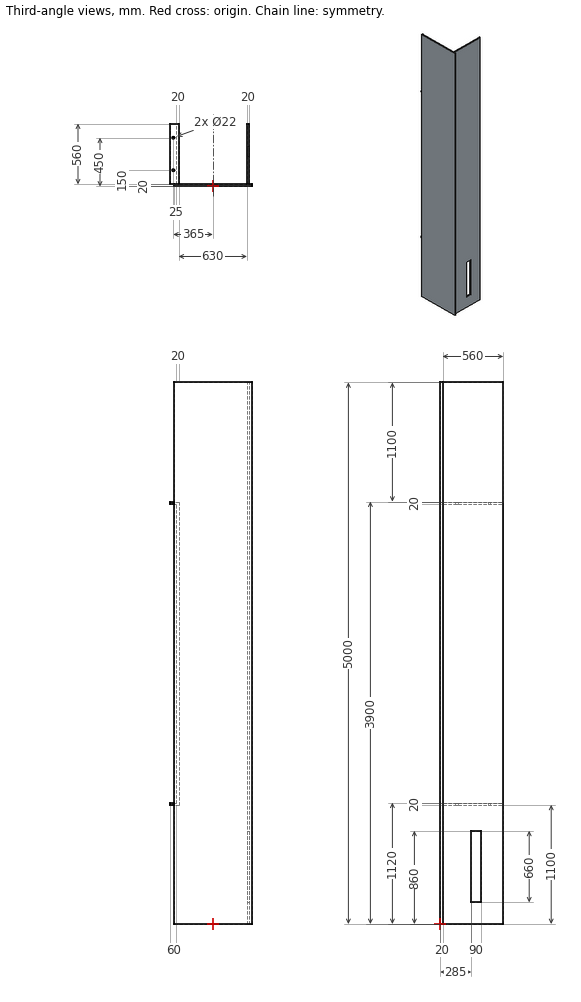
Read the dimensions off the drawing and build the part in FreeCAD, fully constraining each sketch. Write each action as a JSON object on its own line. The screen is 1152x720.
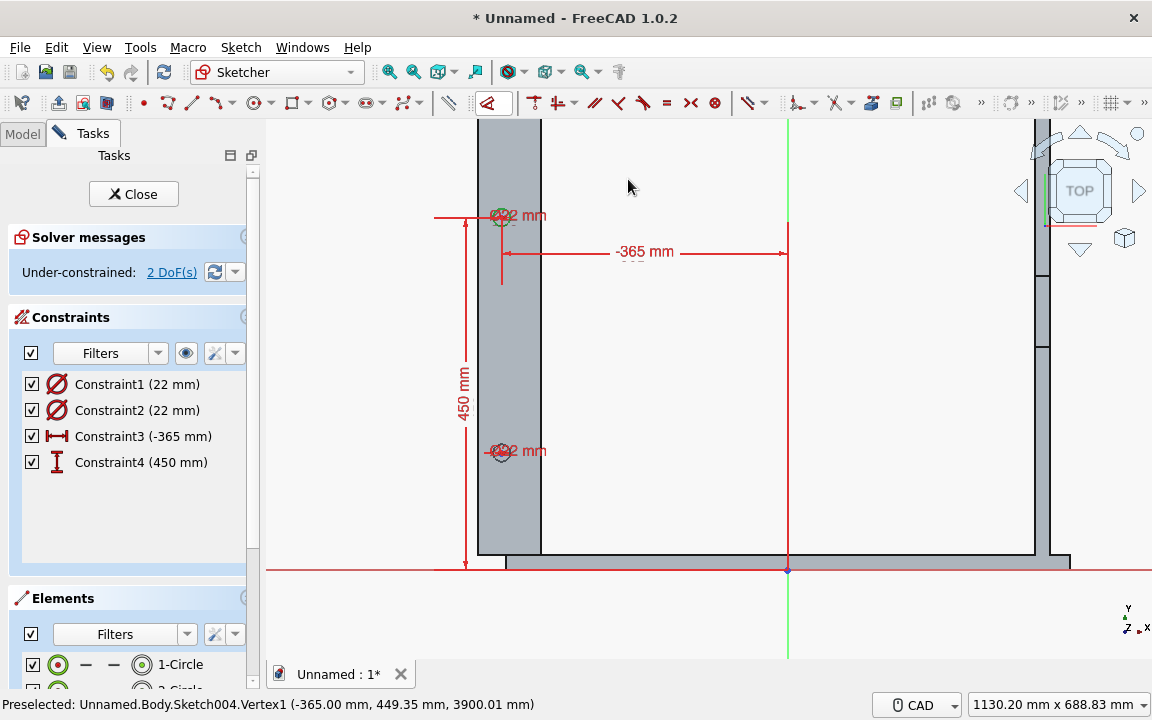
{"action": "left_click", "coordinate": [502, 453]}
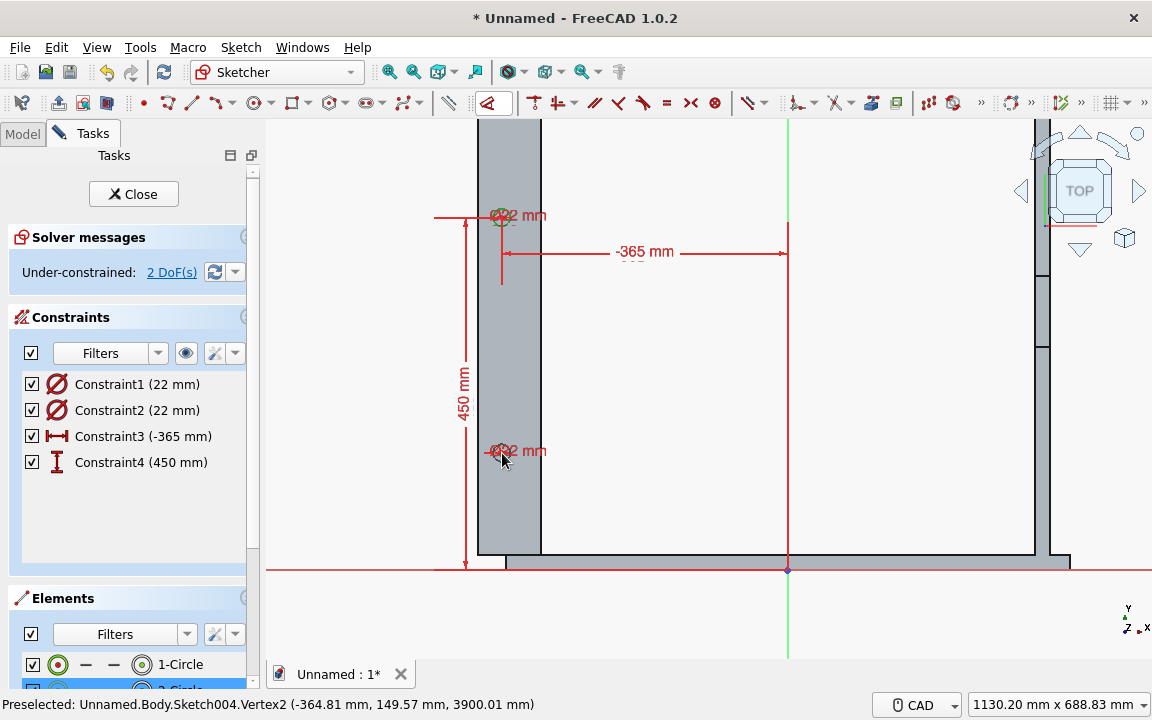
{"action": "key", "text": "l"}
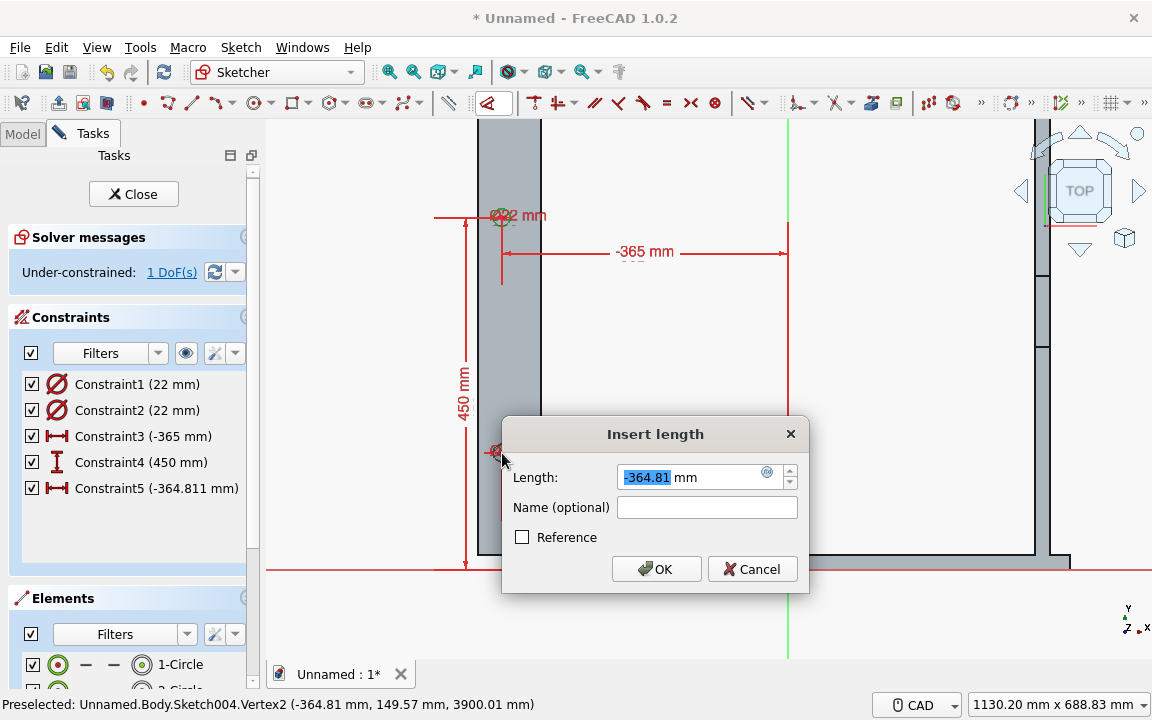
{"action": "type", "text": "-365"}
{"action": "key", "text": "Return"}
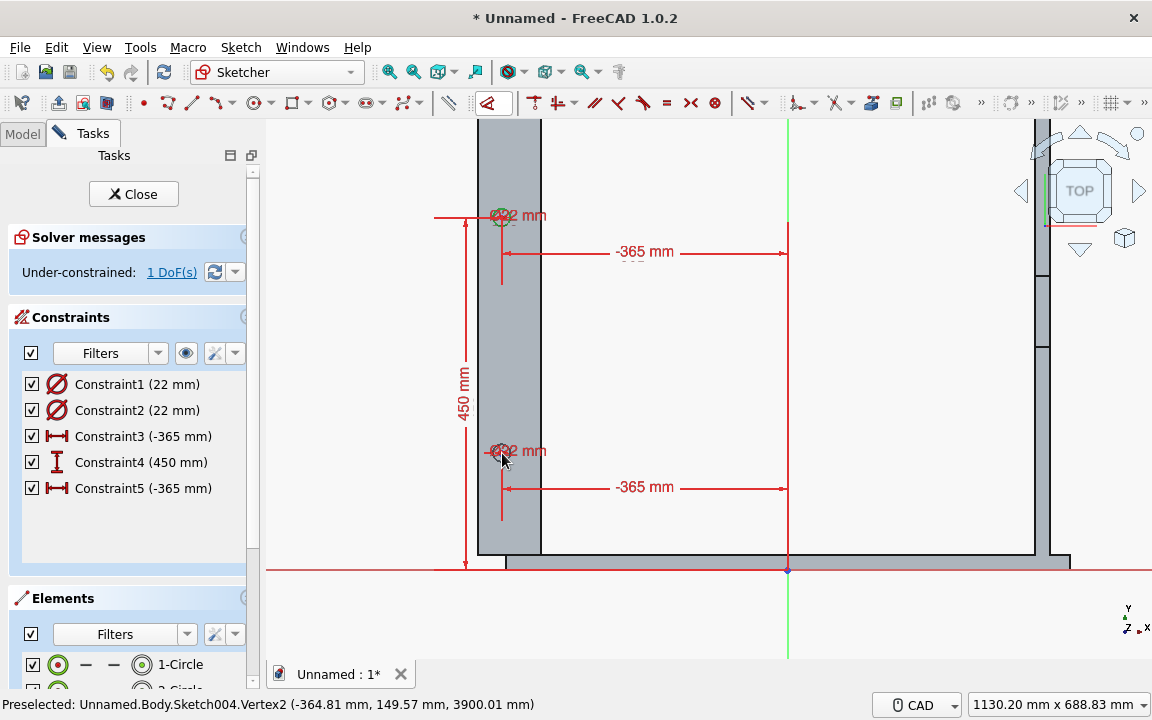
{"action": "left_click", "coordinate": [502, 453]}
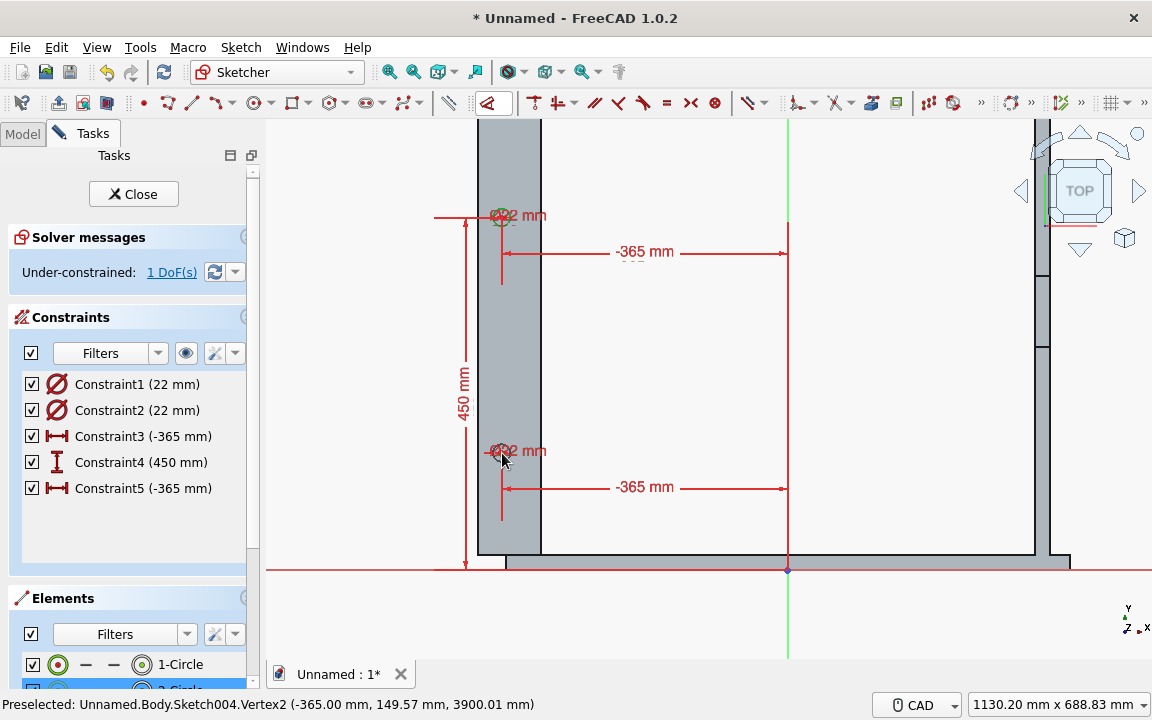
{"action": "left_click", "coordinate": [506, 104]}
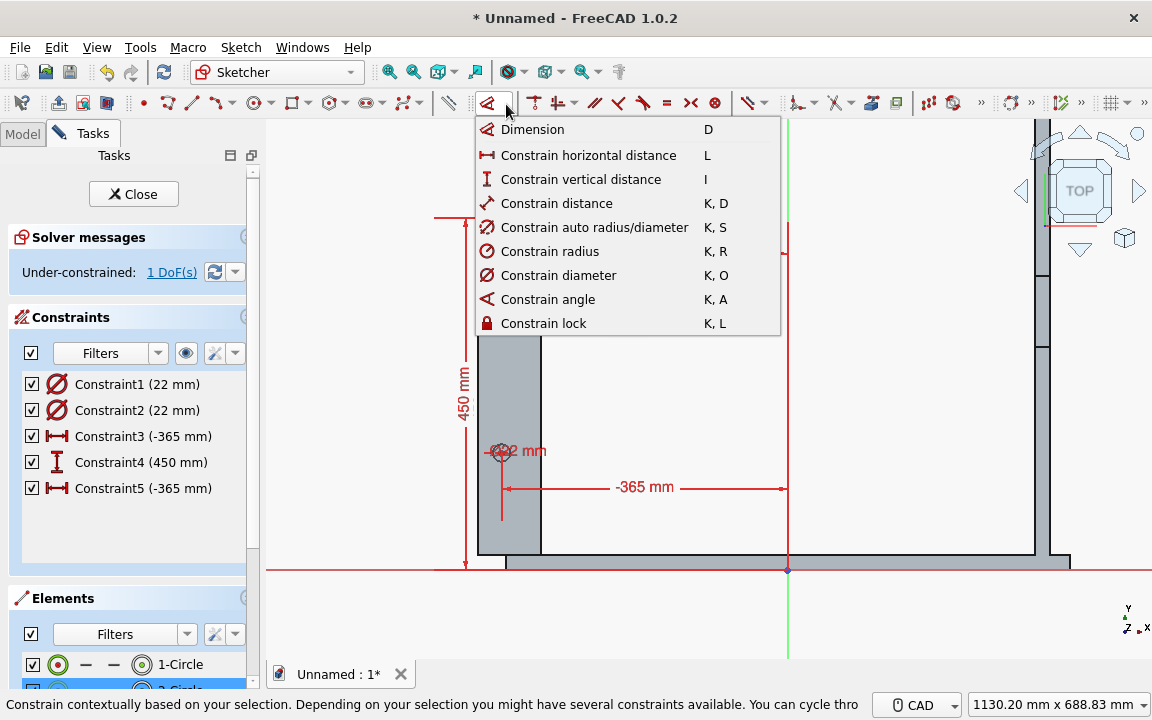
{"action": "left_click", "coordinate": [628, 179]}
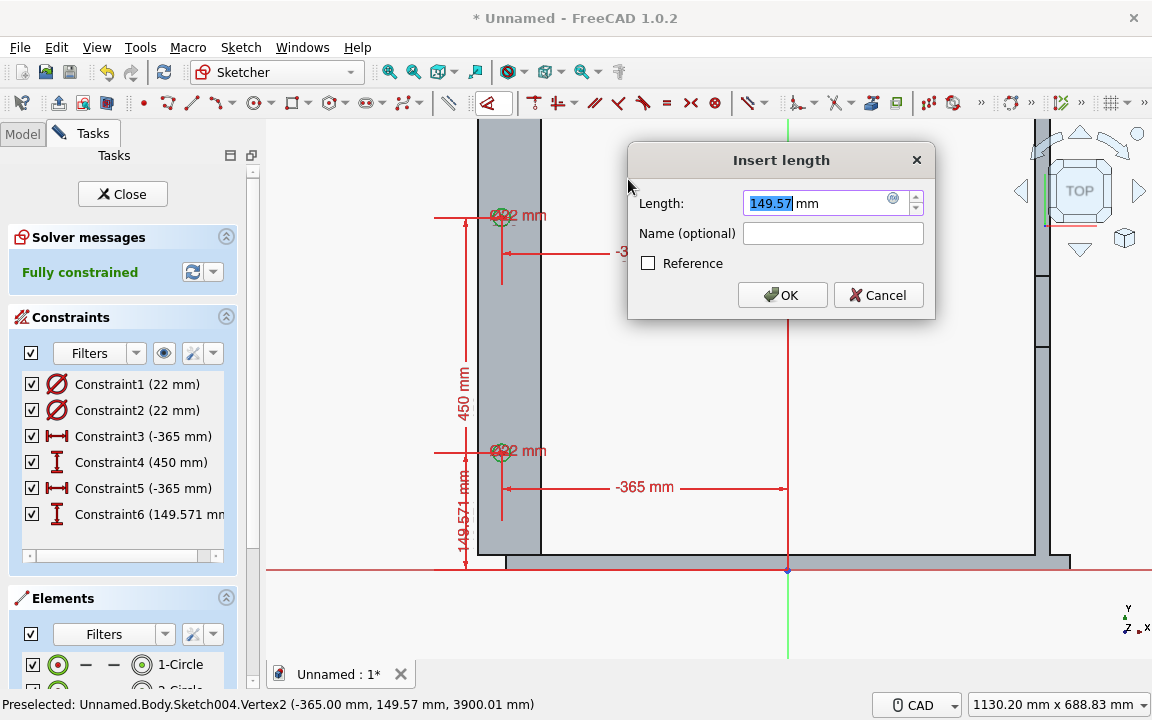
{"action": "type", "text": "150"}
{"action": "key", "text": "Return"}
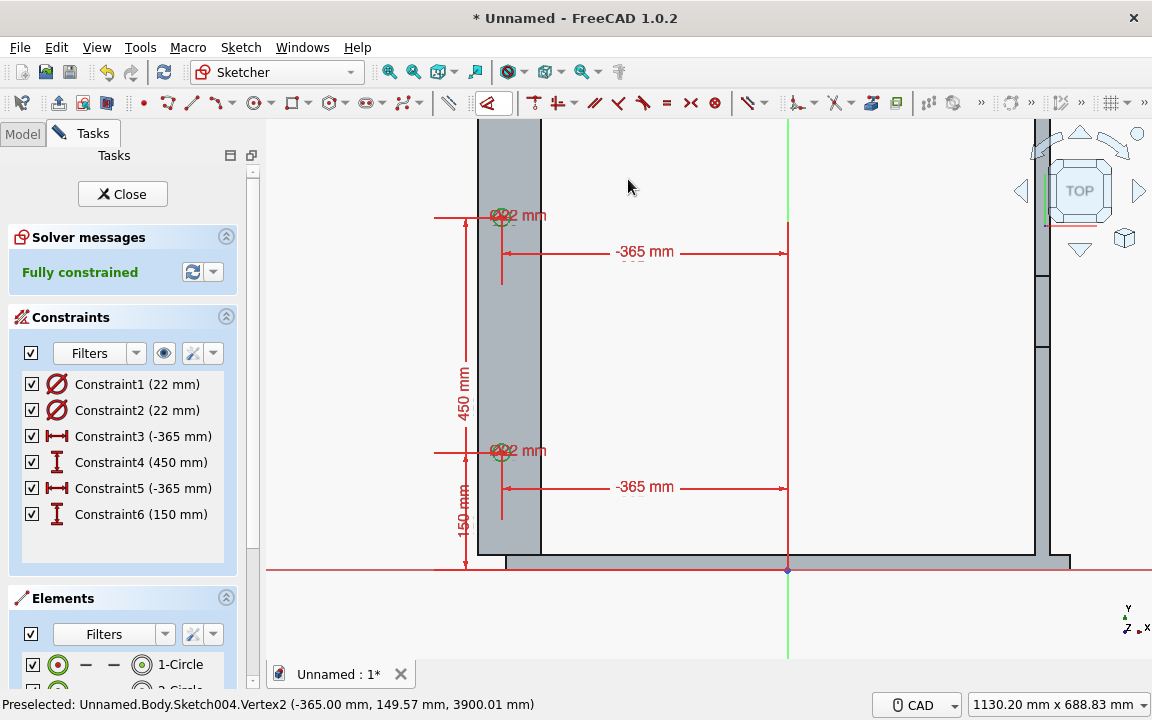
{"action": "left_click", "coordinate": [123, 194]}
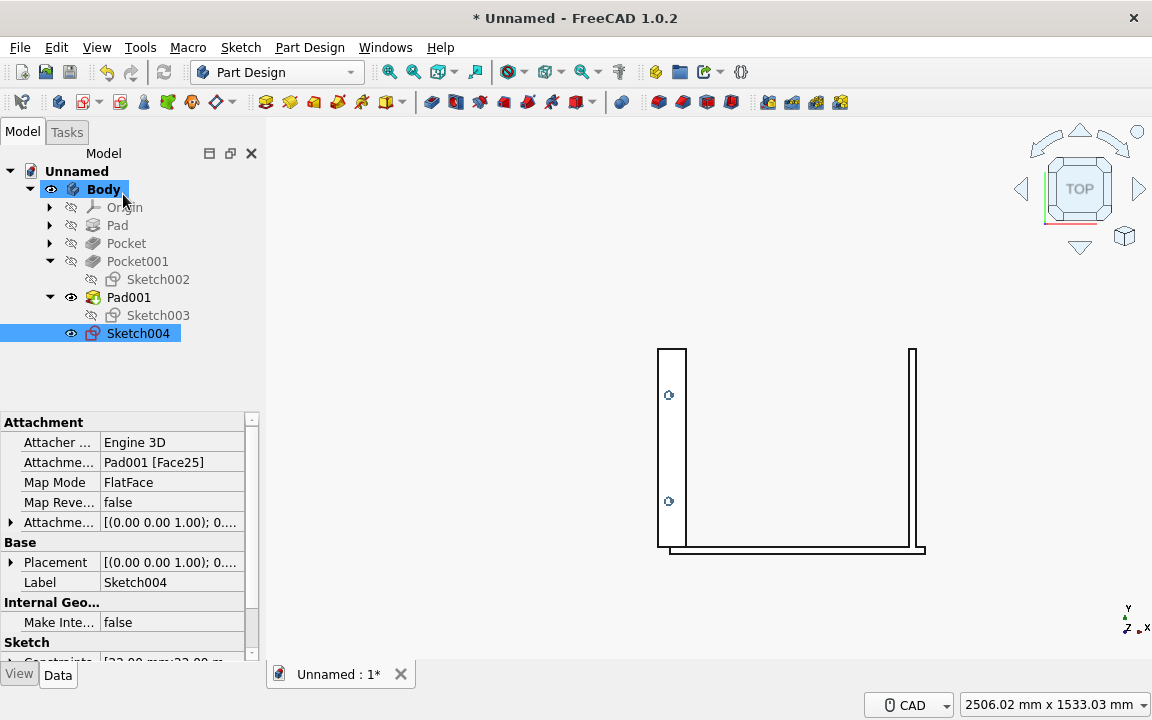
{"action": "left_click", "coordinate": [432, 102]}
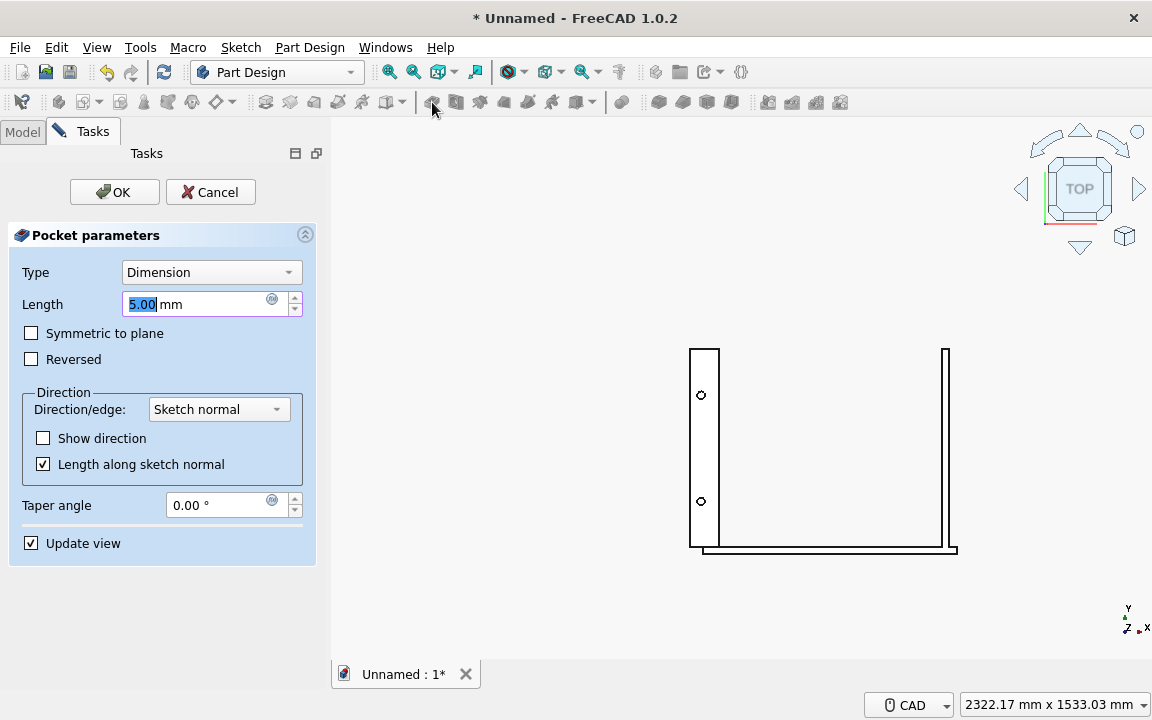
{"action": "left_click", "coordinate": [212, 272]}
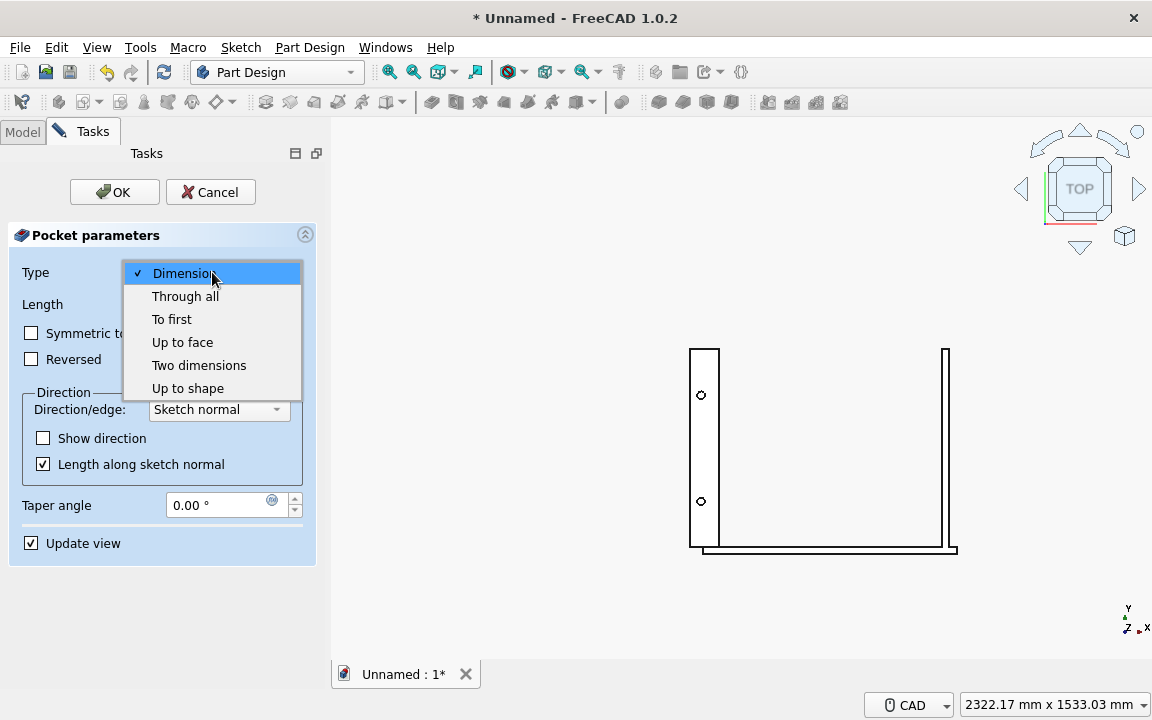
{"action": "left_click", "coordinate": [212, 296]}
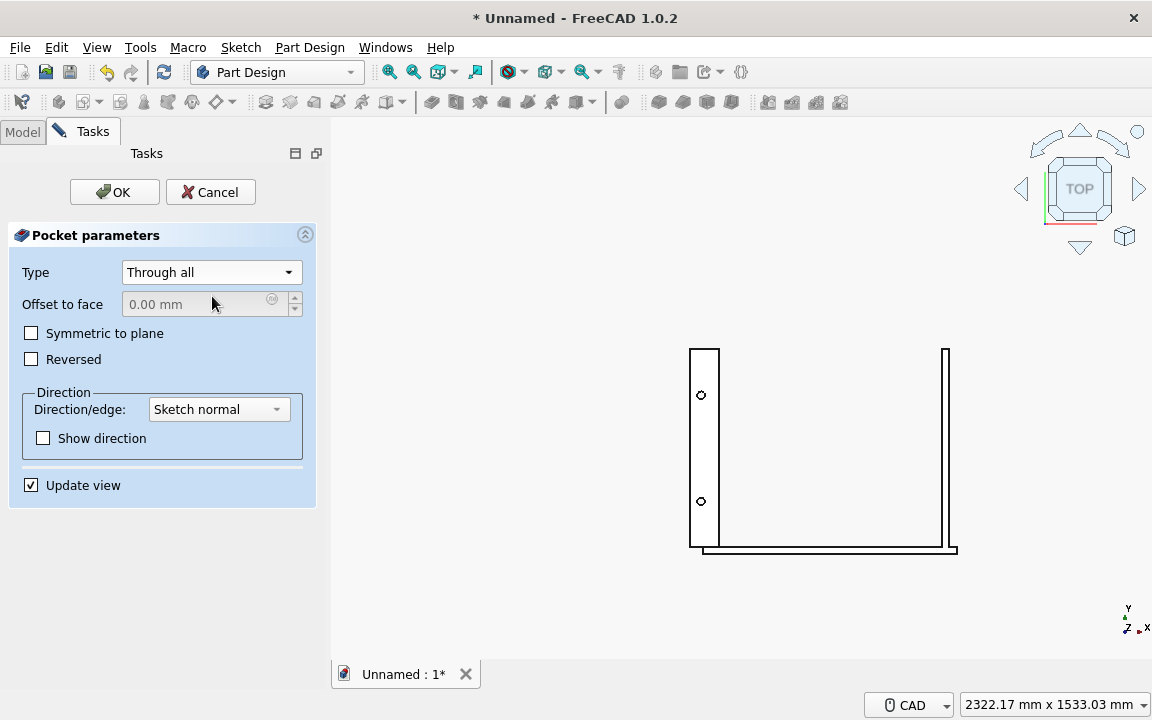
{"action": "left_click", "coordinate": [115, 192]}